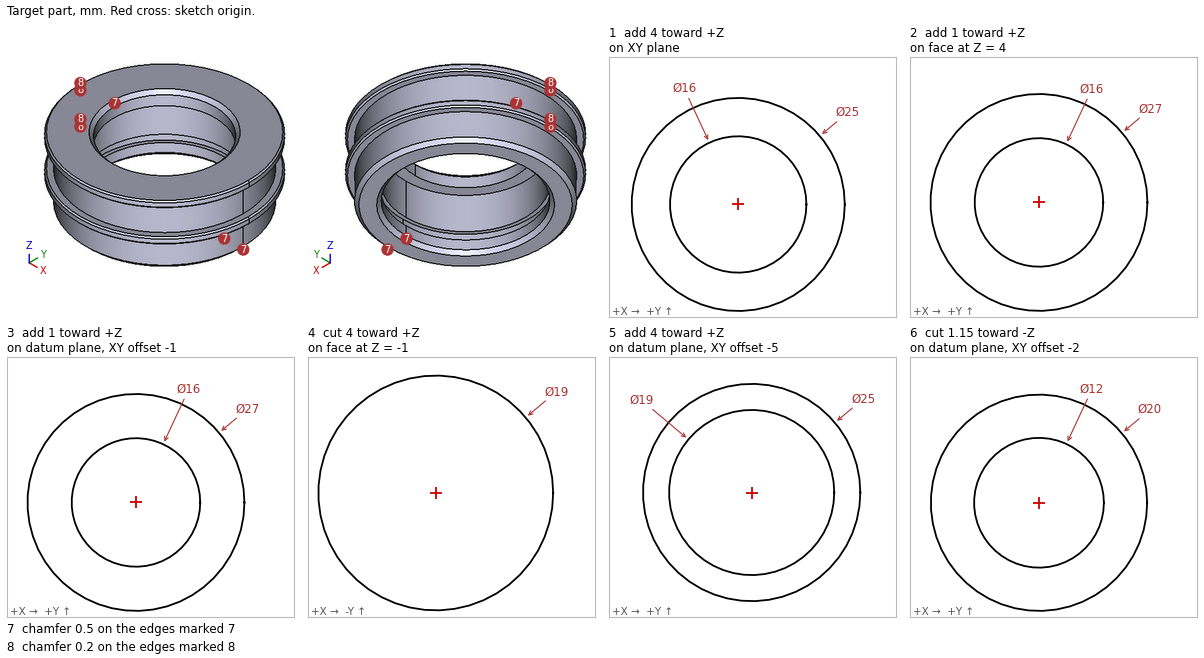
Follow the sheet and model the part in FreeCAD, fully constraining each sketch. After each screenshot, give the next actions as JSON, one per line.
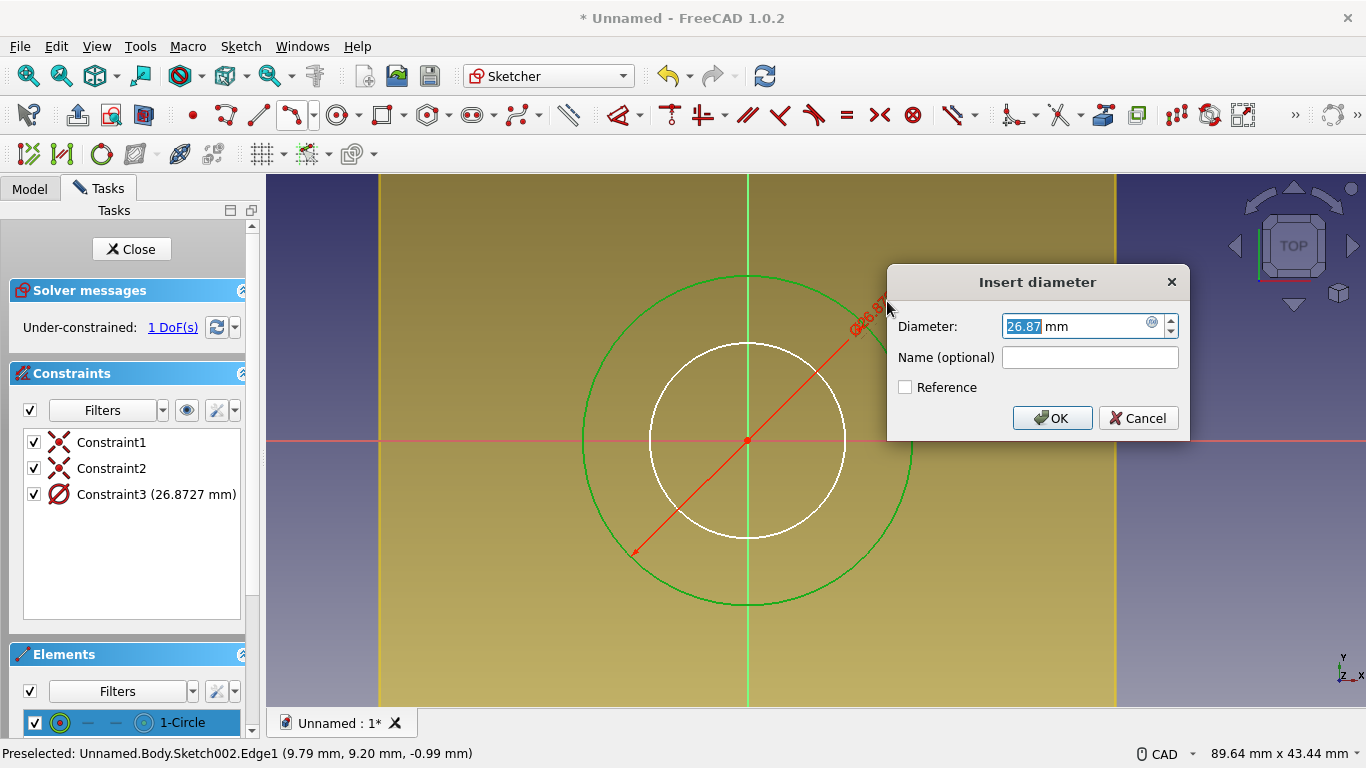
{"action": "type", "text": "27"}
{"action": "key", "text": "Return"}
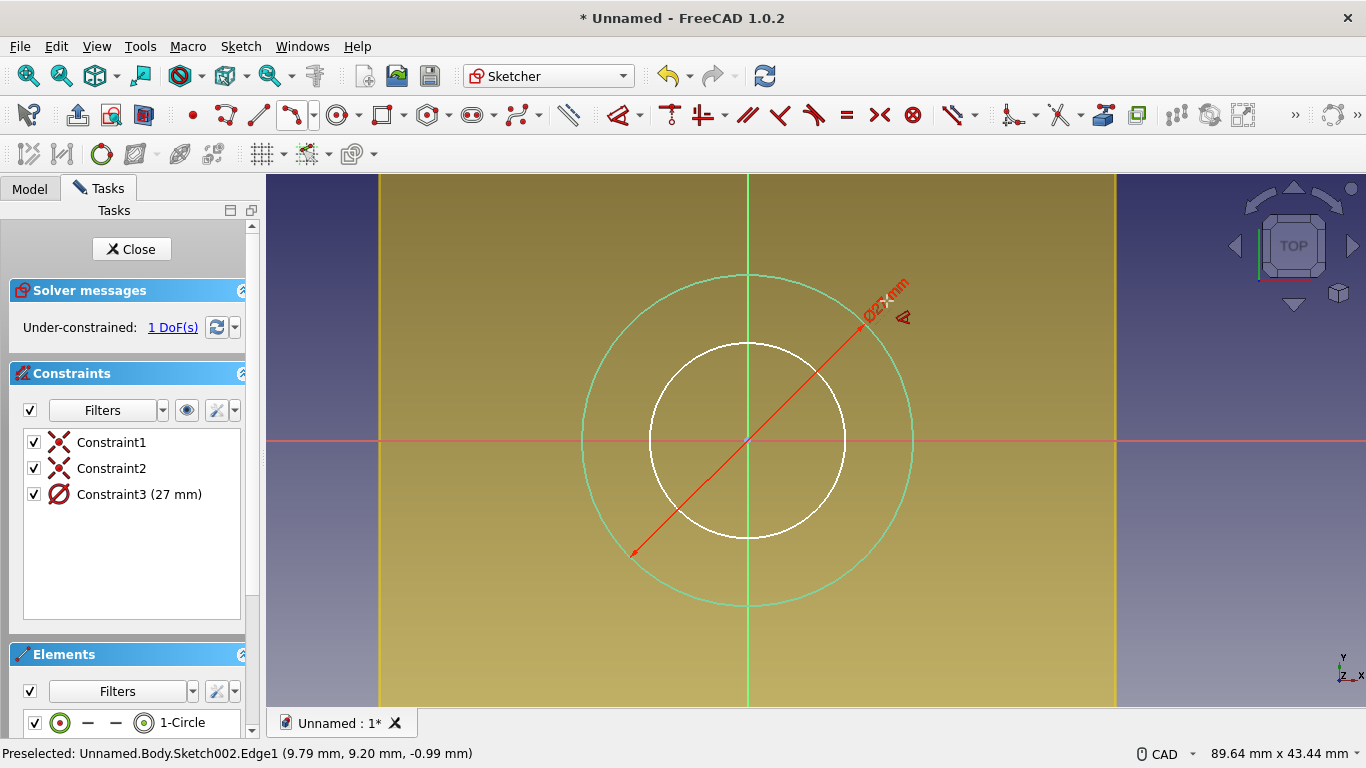
{"action": "left_click", "coordinate": [816, 371]}
{"action": "left_click", "coordinate": [838, 348]}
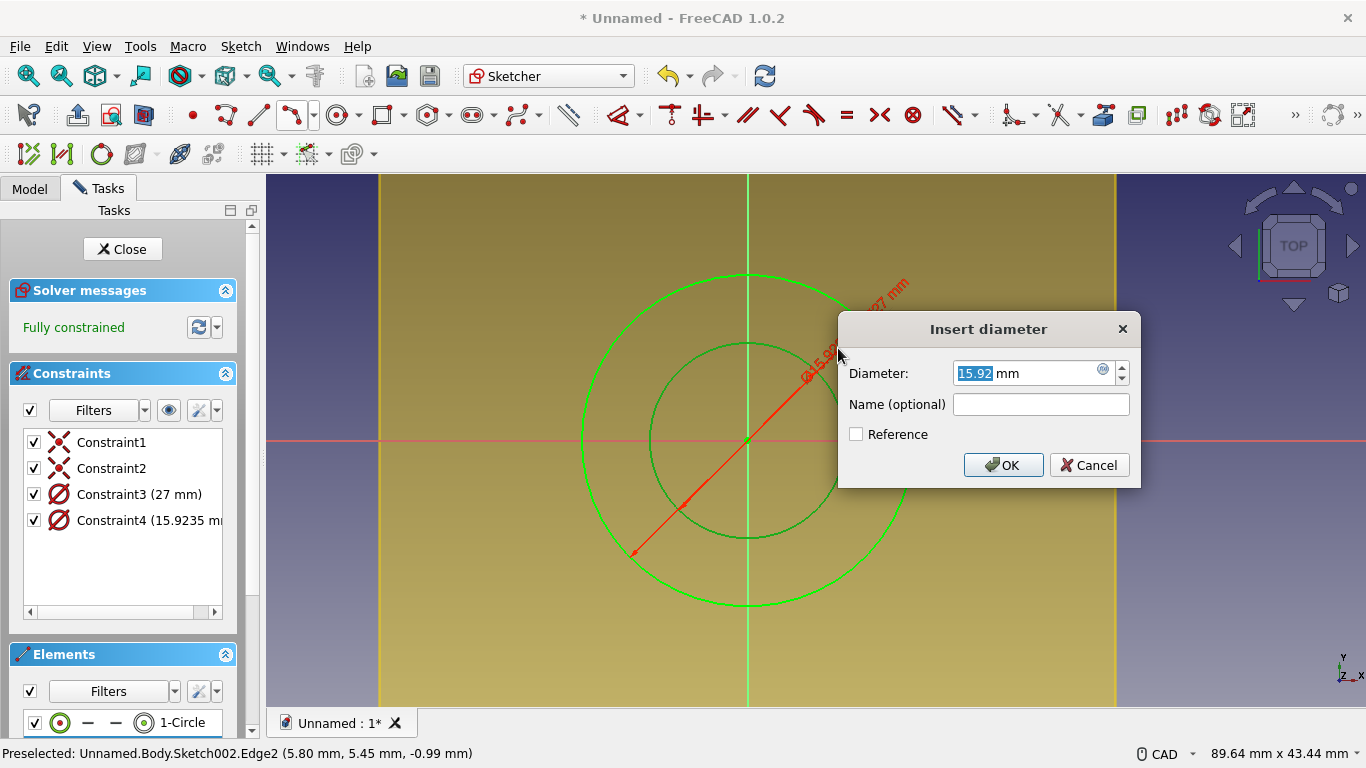
{"action": "type", "text": "16"}
{"action": "key", "text": "Return"}
{"action": "key", "text": "Escape"}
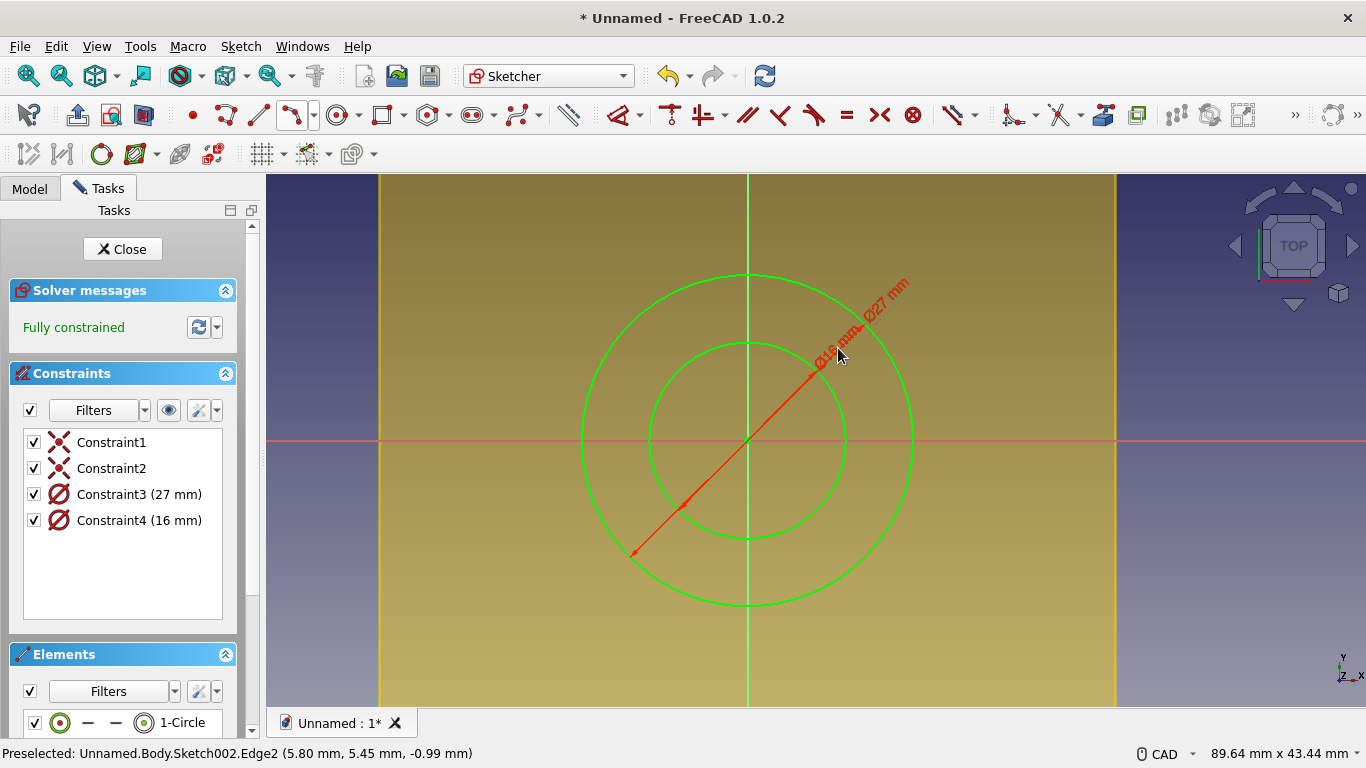
{"action": "left_click", "coordinate": [123, 249]}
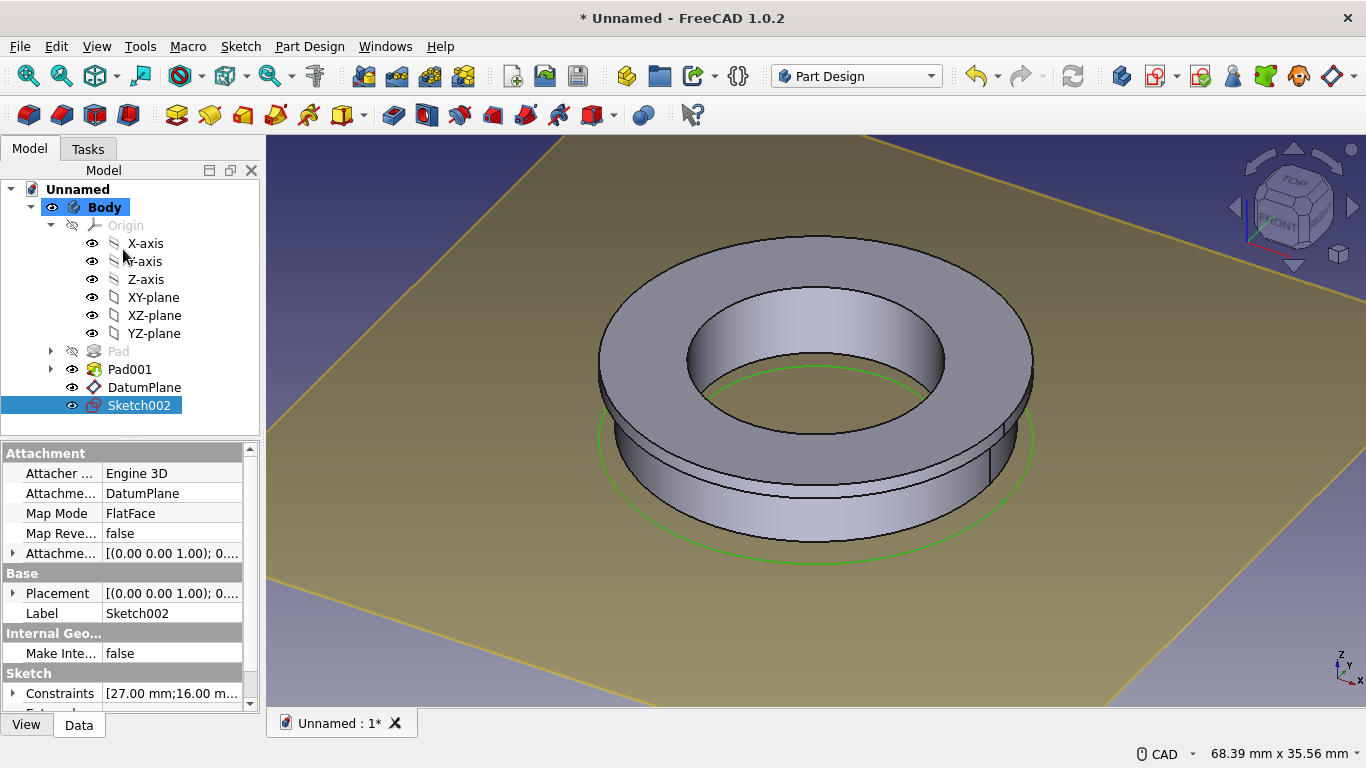
{"action": "left_click", "coordinate": [177, 116]}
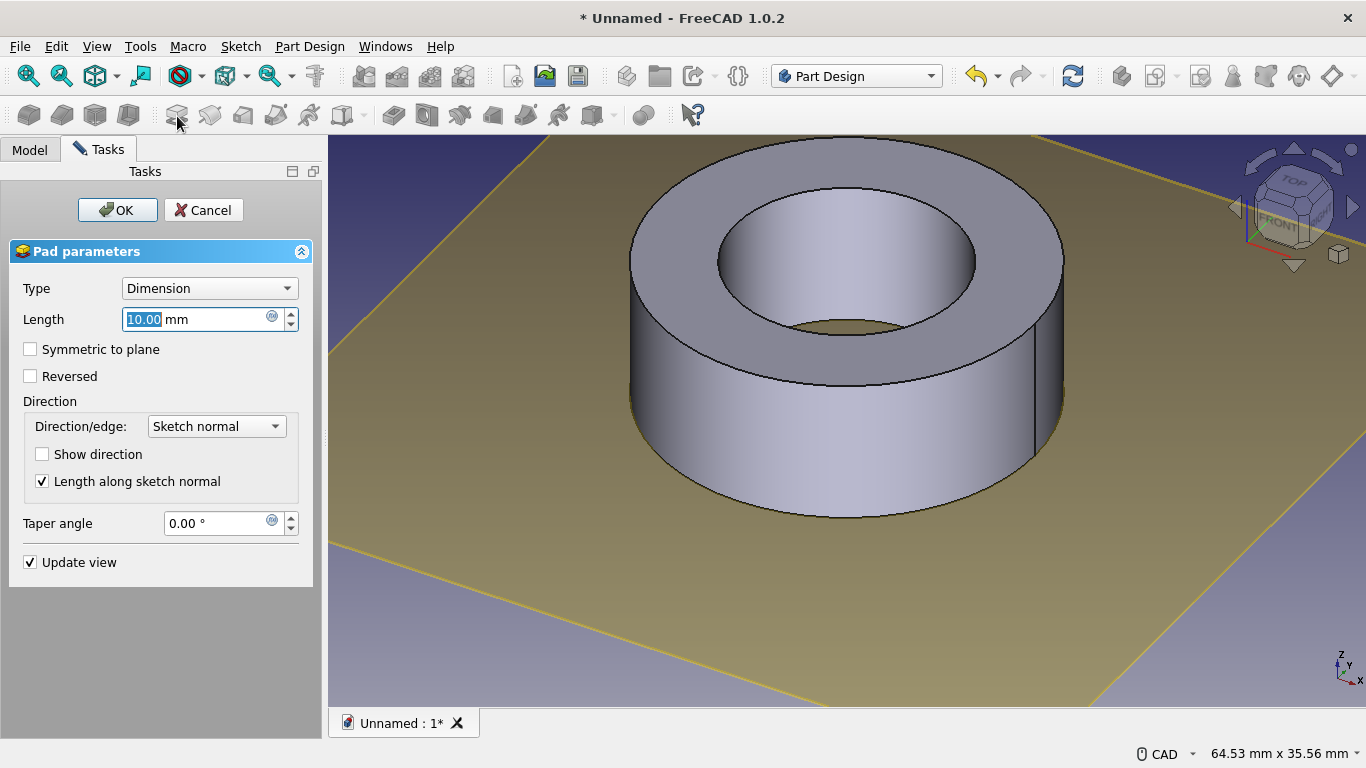
{"action": "type", "text": "1"}
{"action": "key", "text": "Tab"}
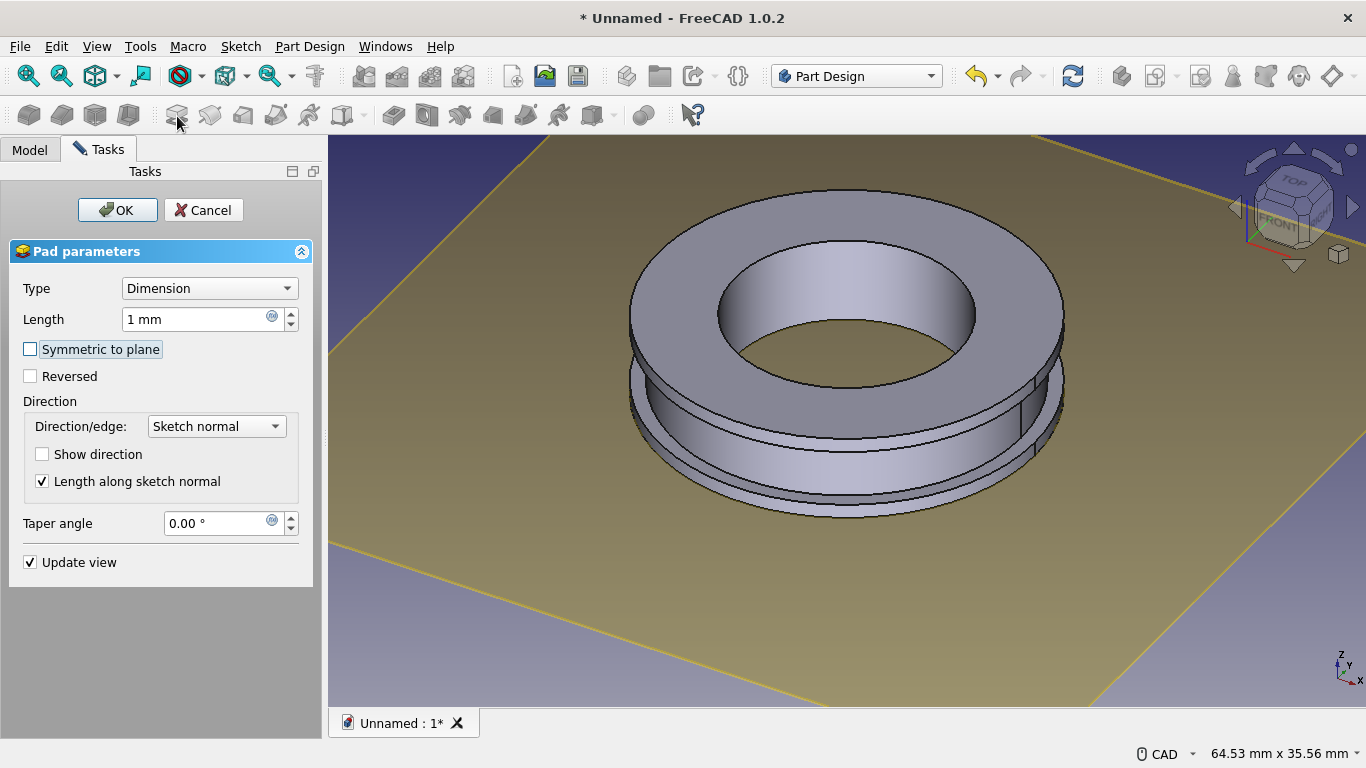
{"action": "left_click", "coordinate": [118, 210]}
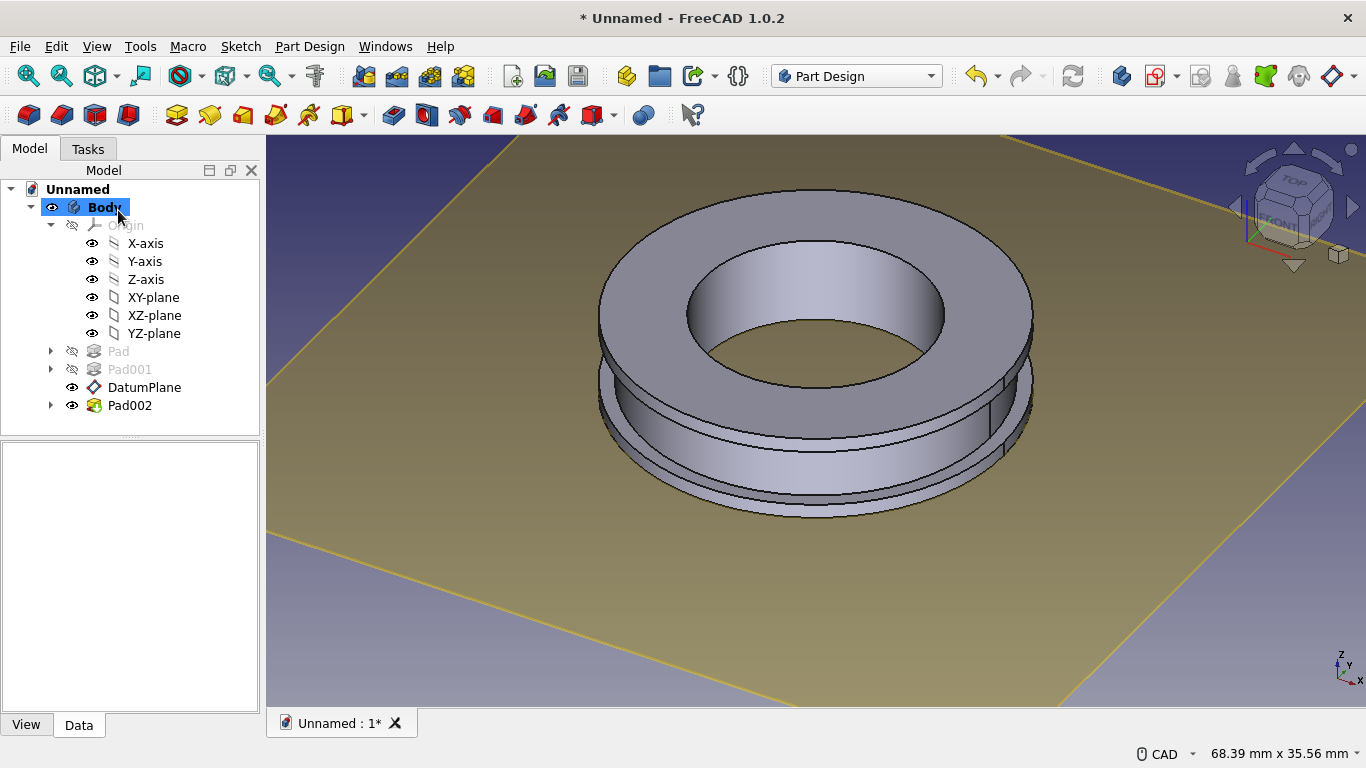
{"action": "left_click", "coordinate": [117, 387]}
{"action": "key", "text": "space"}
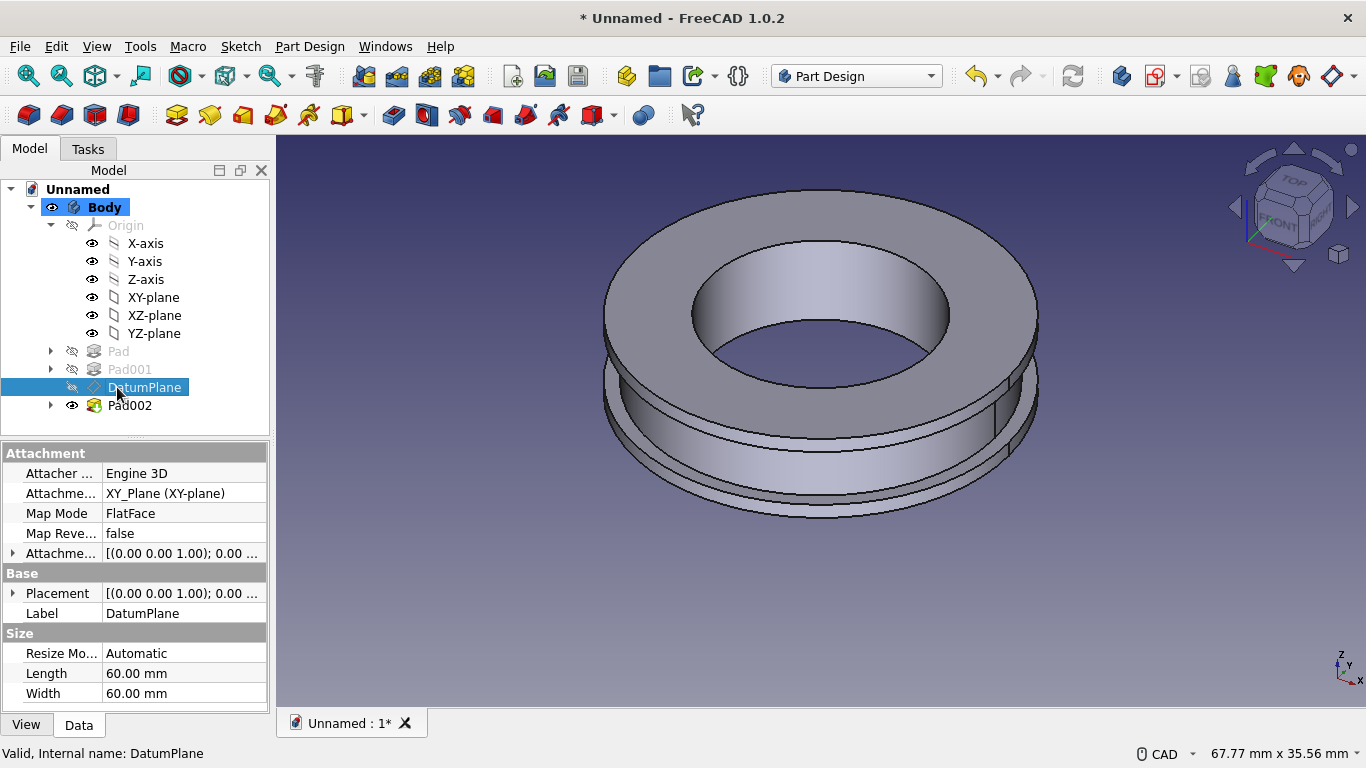
{"action": "key", "text": "5"}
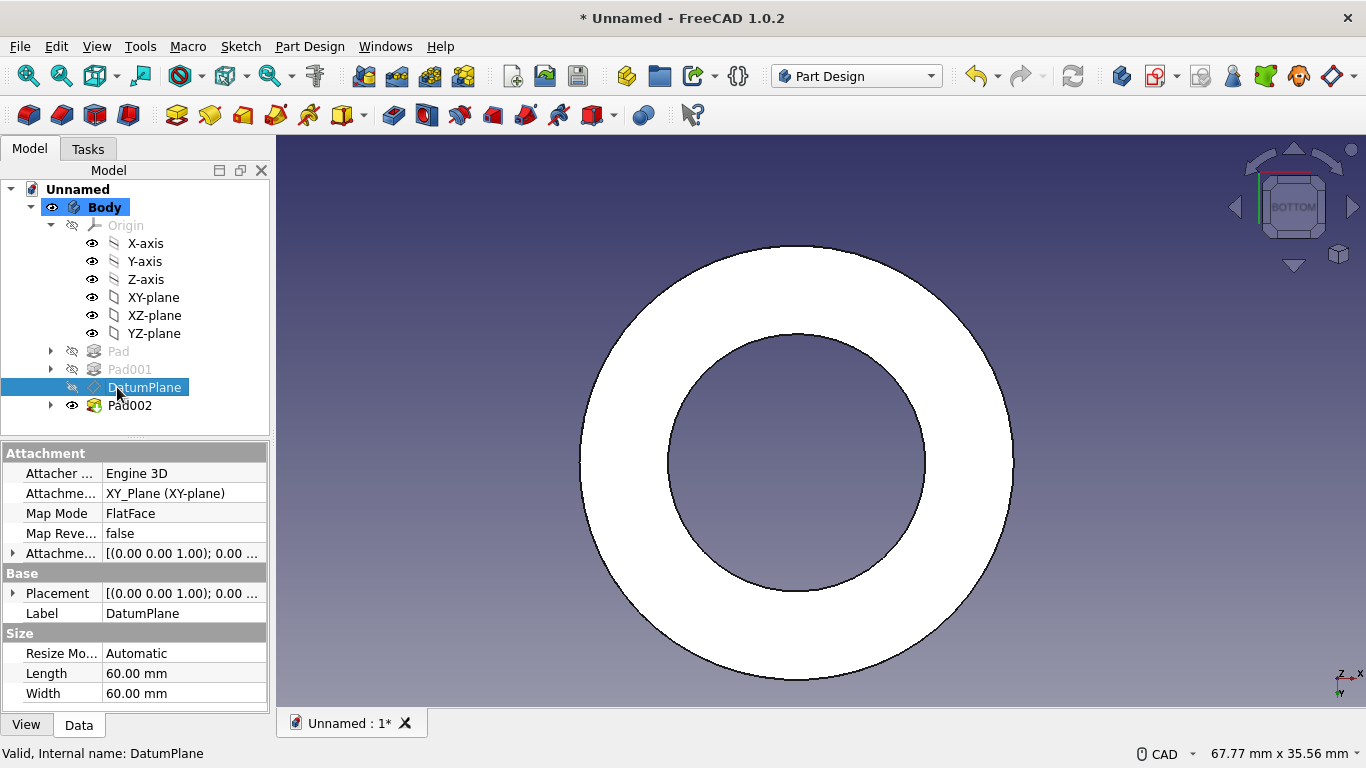
{"action": "left_click", "coordinate": [673, 338]}